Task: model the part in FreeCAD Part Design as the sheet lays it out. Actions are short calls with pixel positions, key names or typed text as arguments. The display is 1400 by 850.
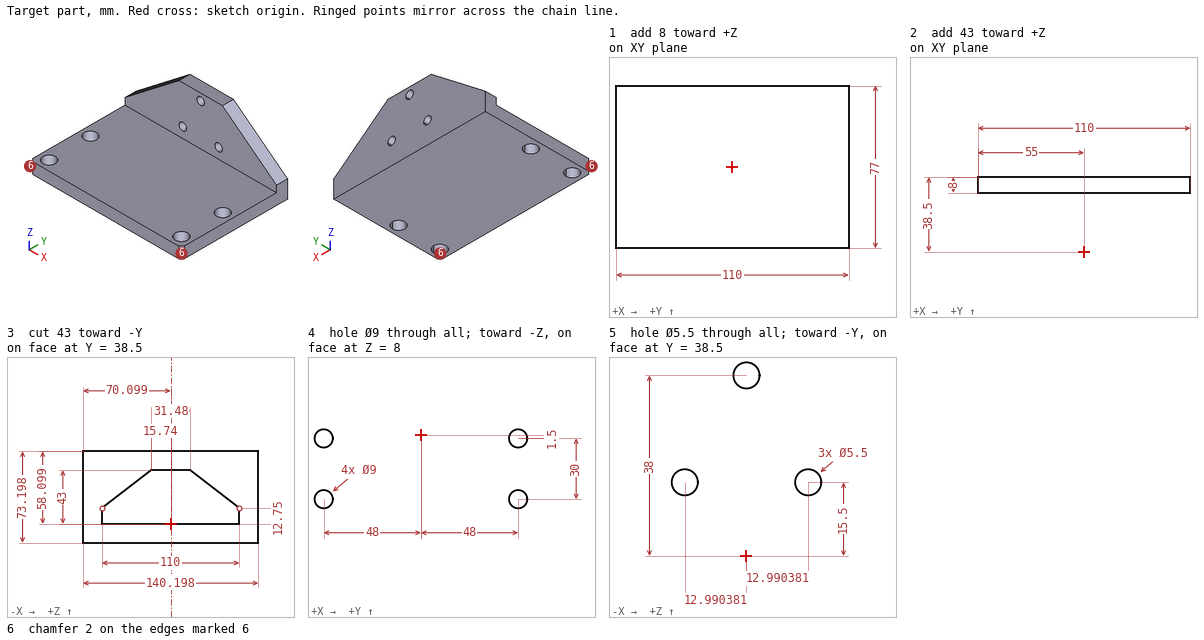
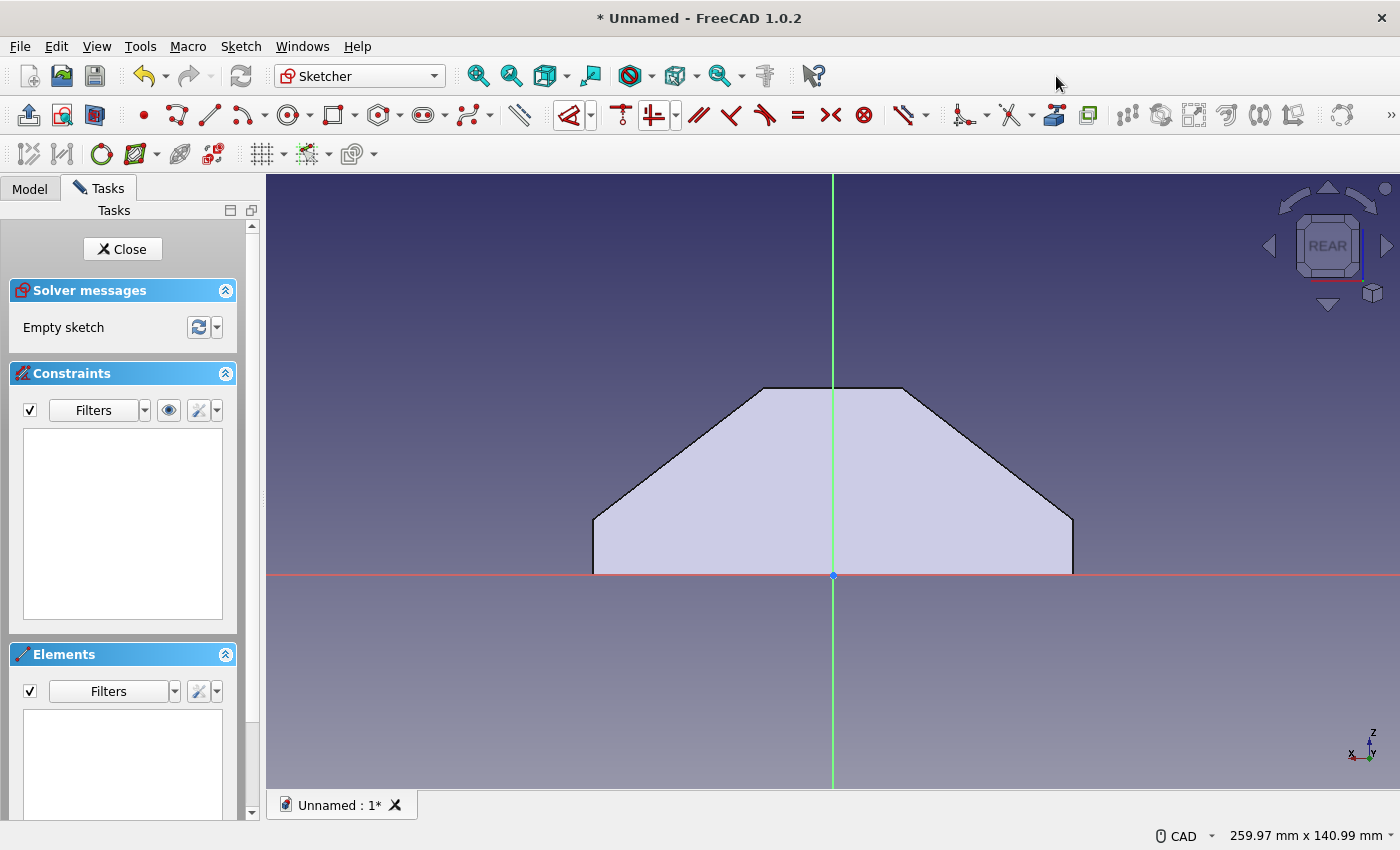
scroll(889, 490, up, 4)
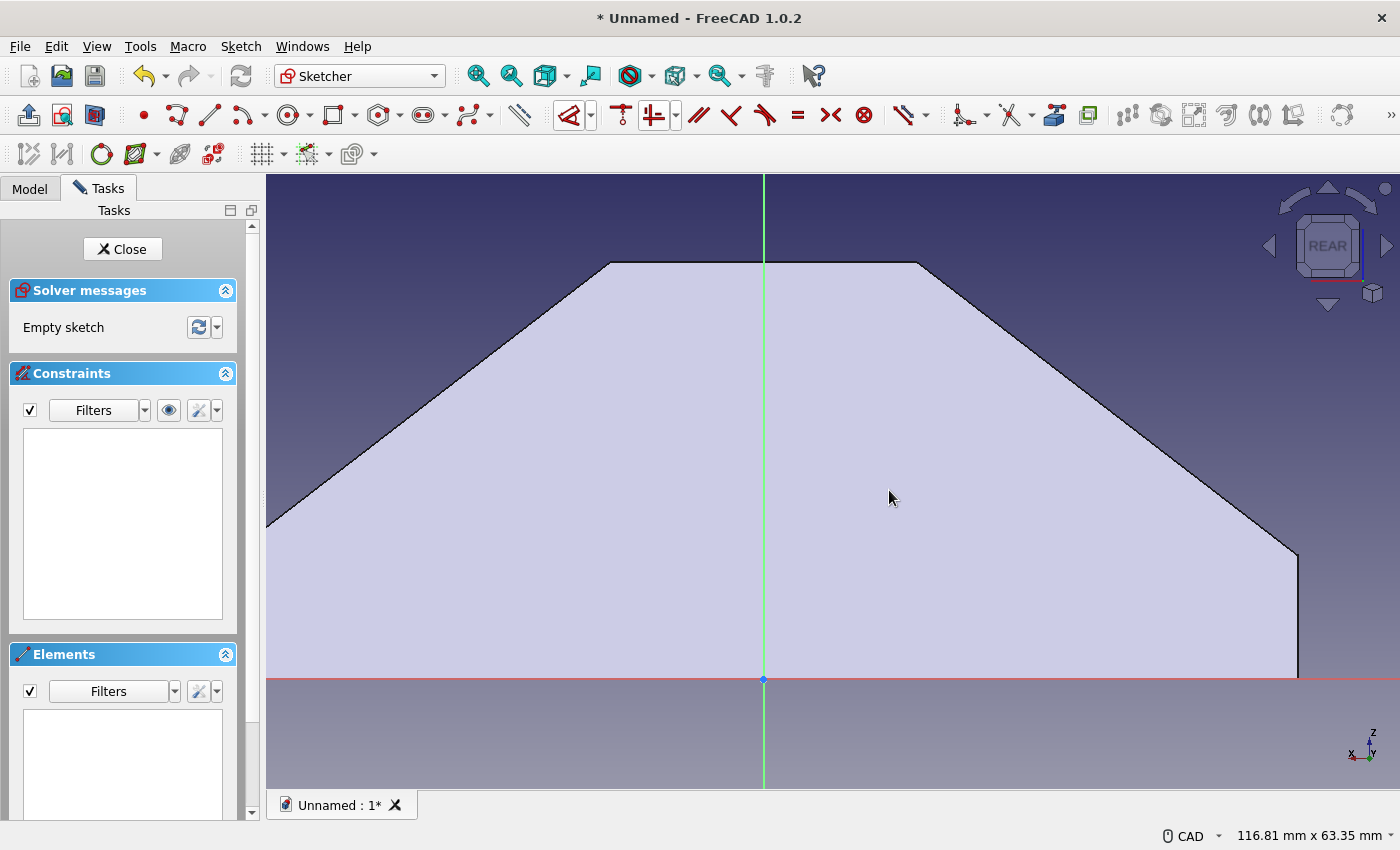
click(288, 116)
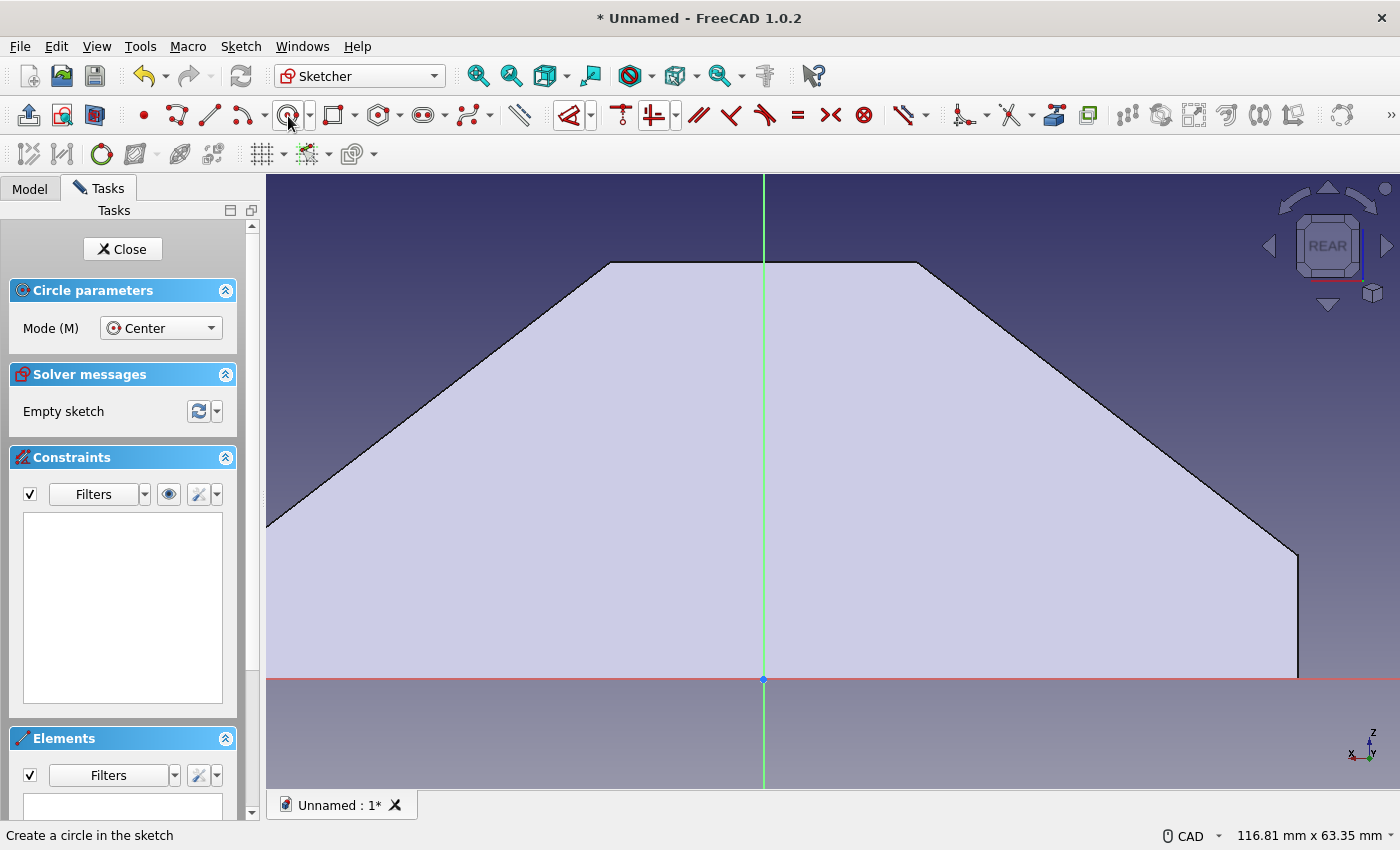
click(890, 529)
click(909, 510)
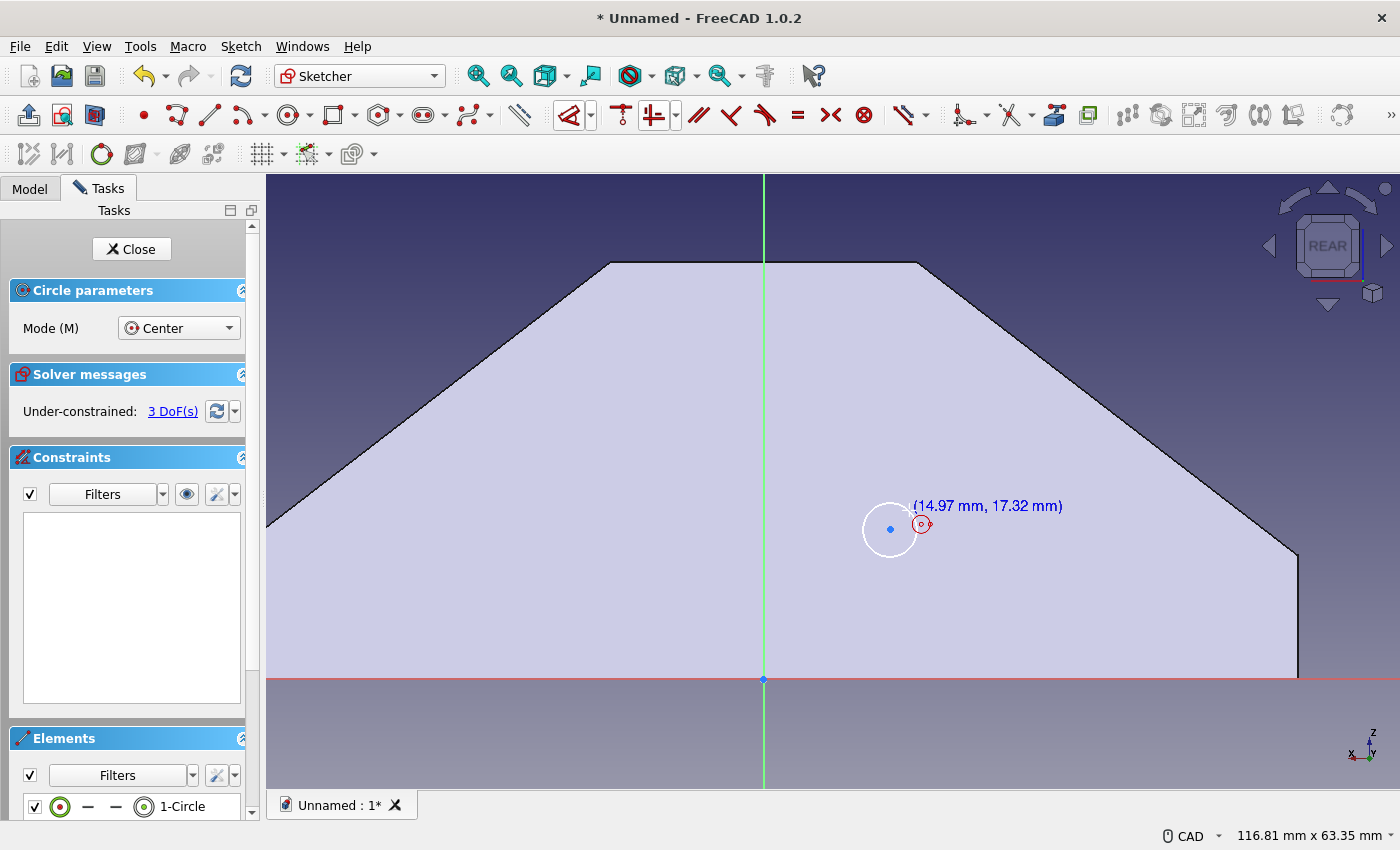
click(638, 529)
click(656, 510)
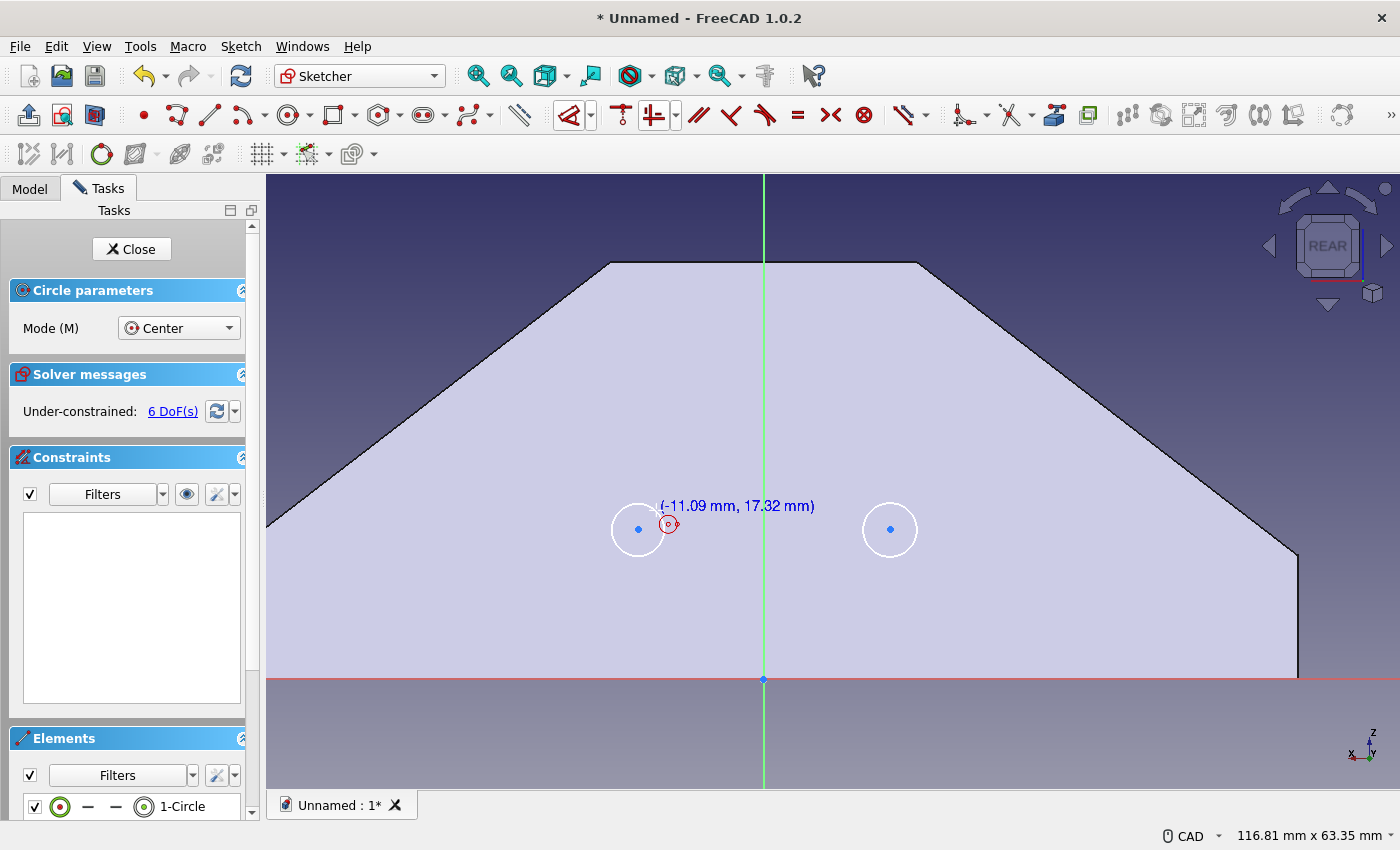
click(764, 310)
click(783, 291)
key(Escape)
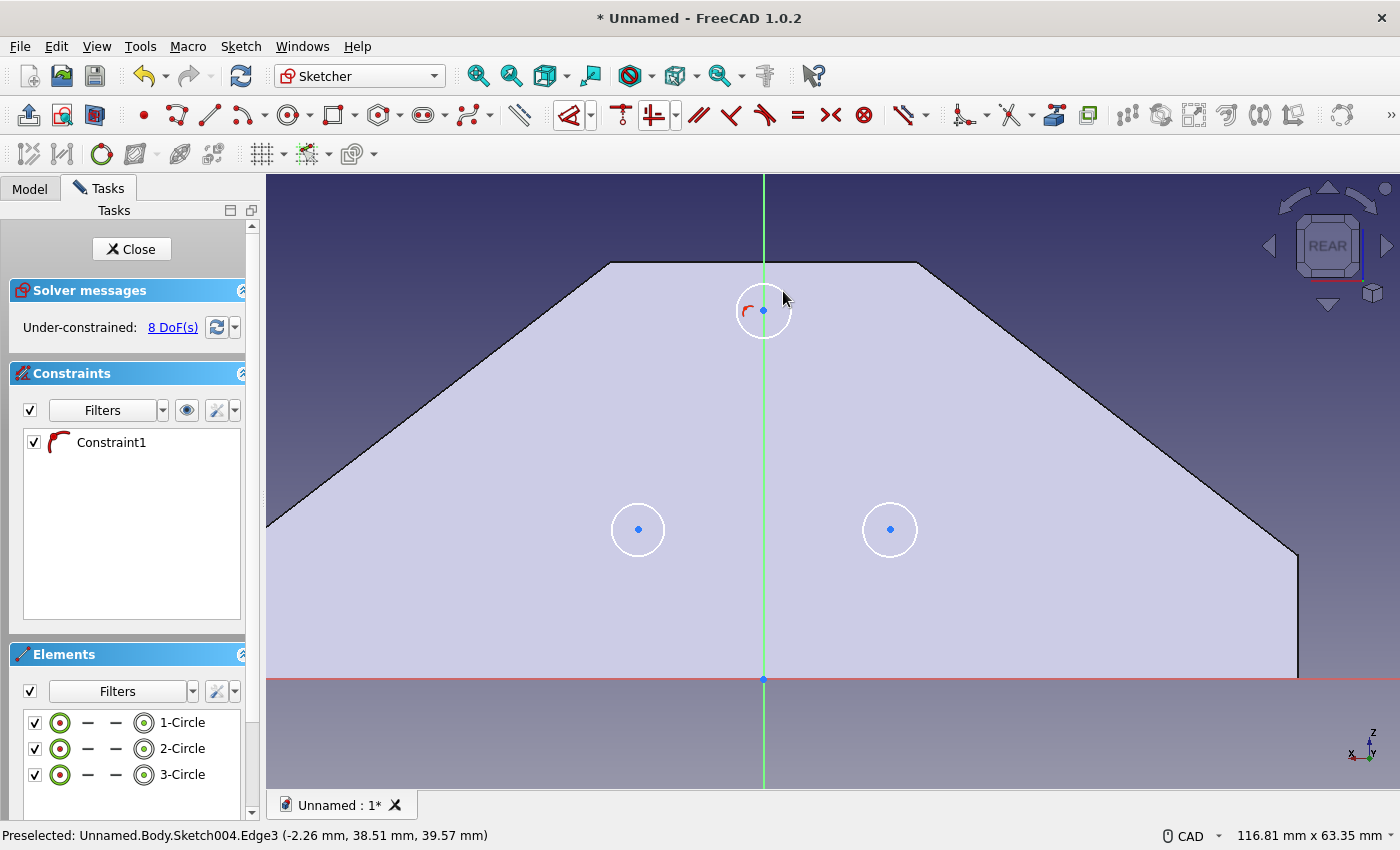
click(909, 511)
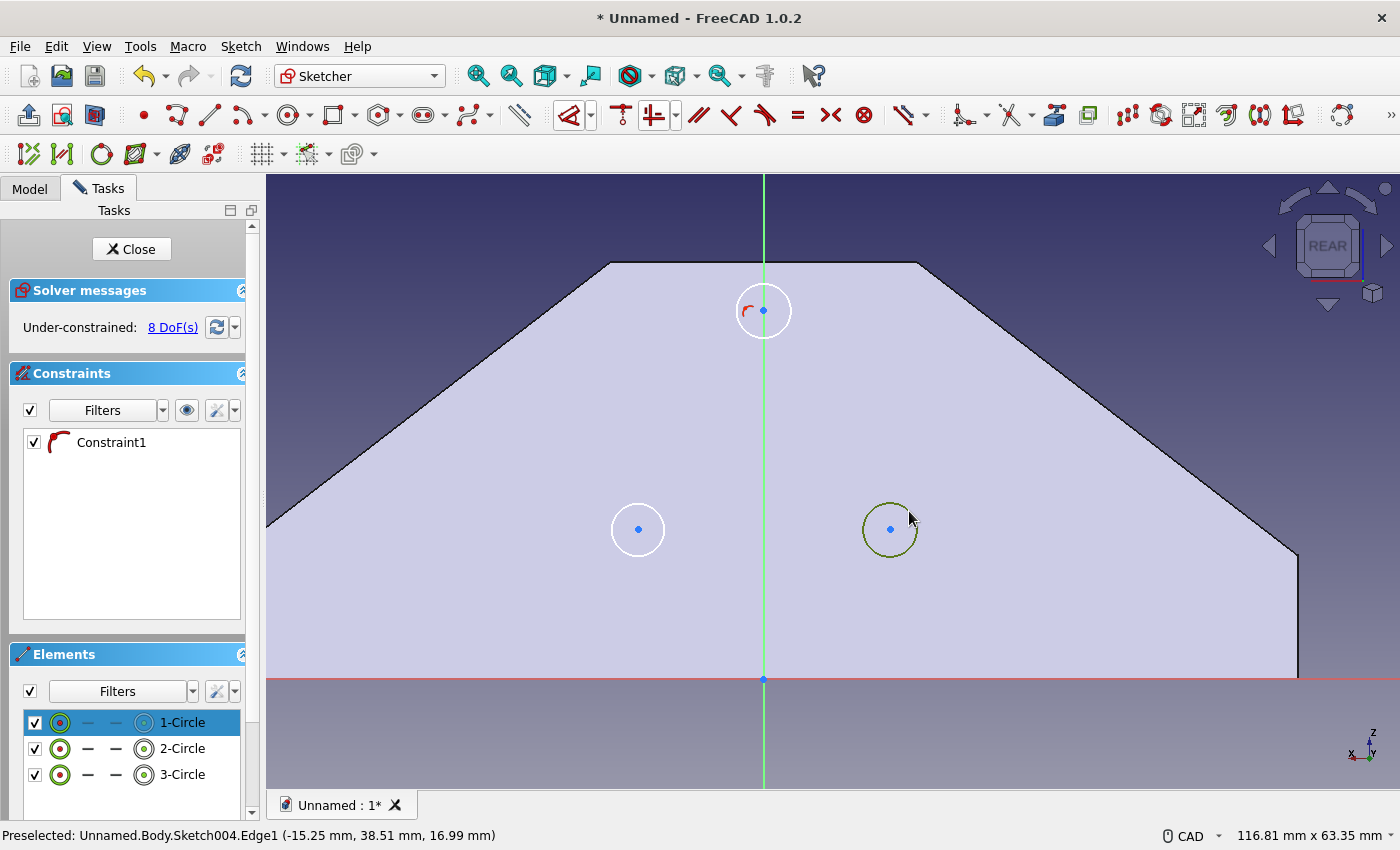
click(656, 511)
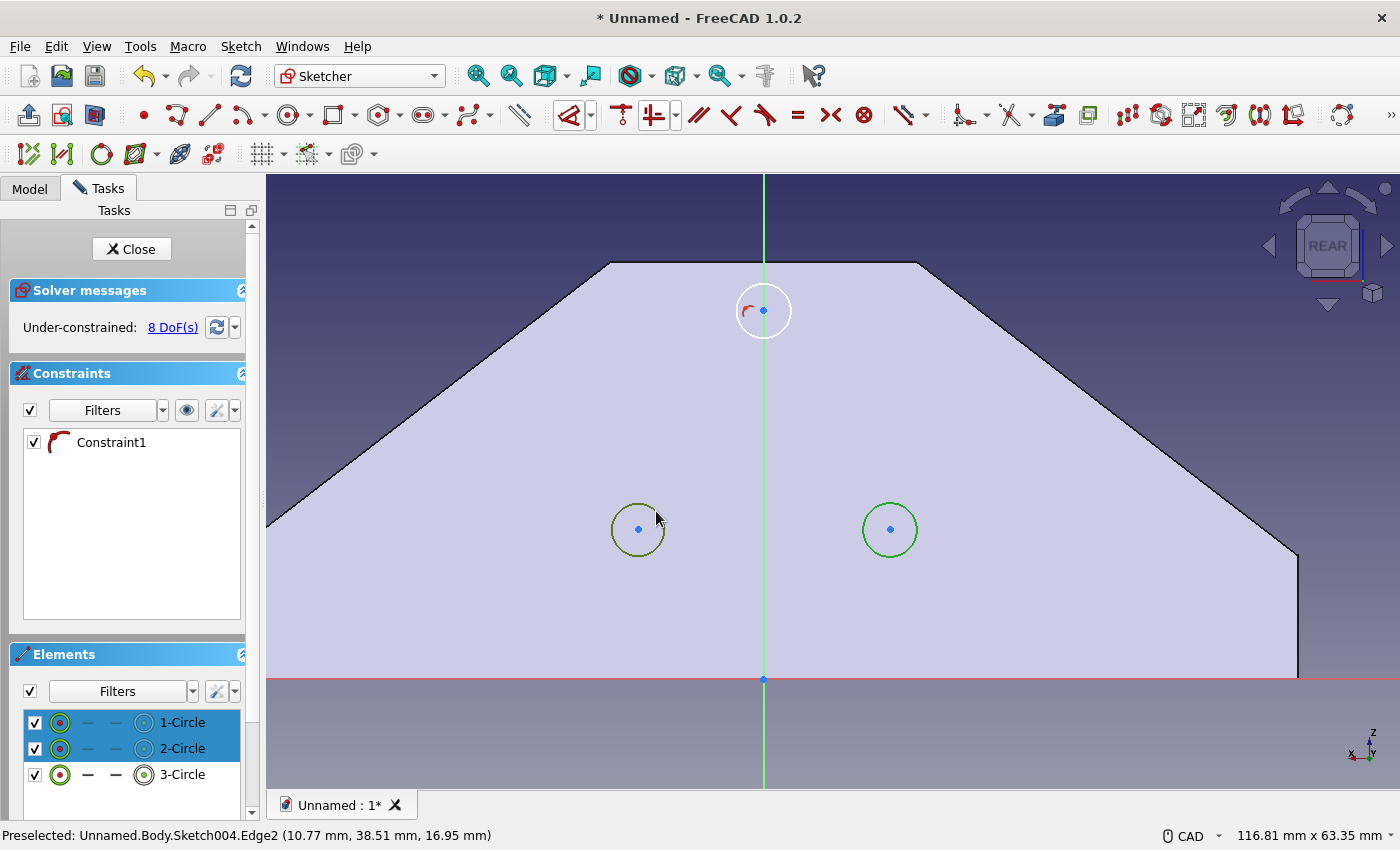
click(783, 292)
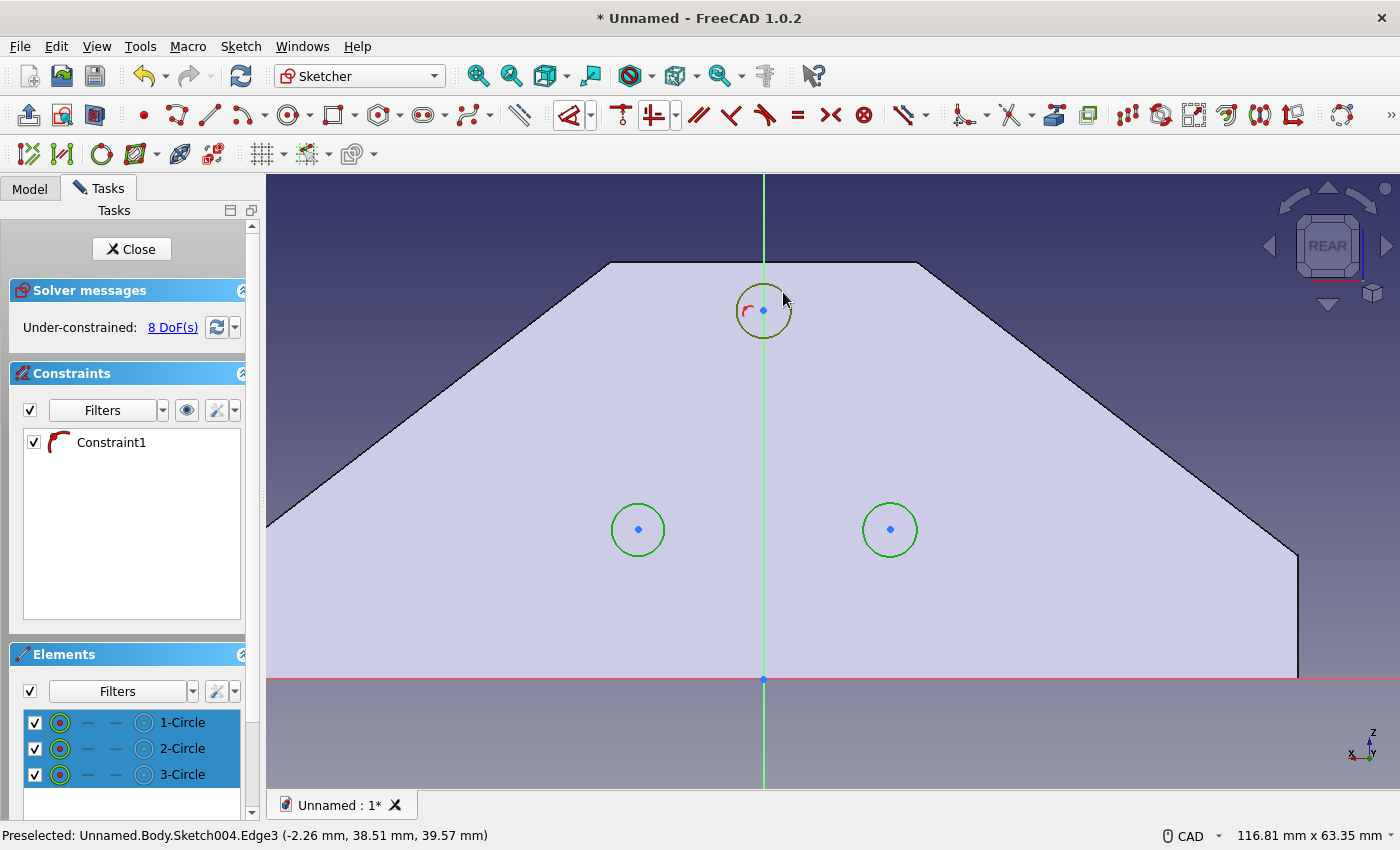
key(e)